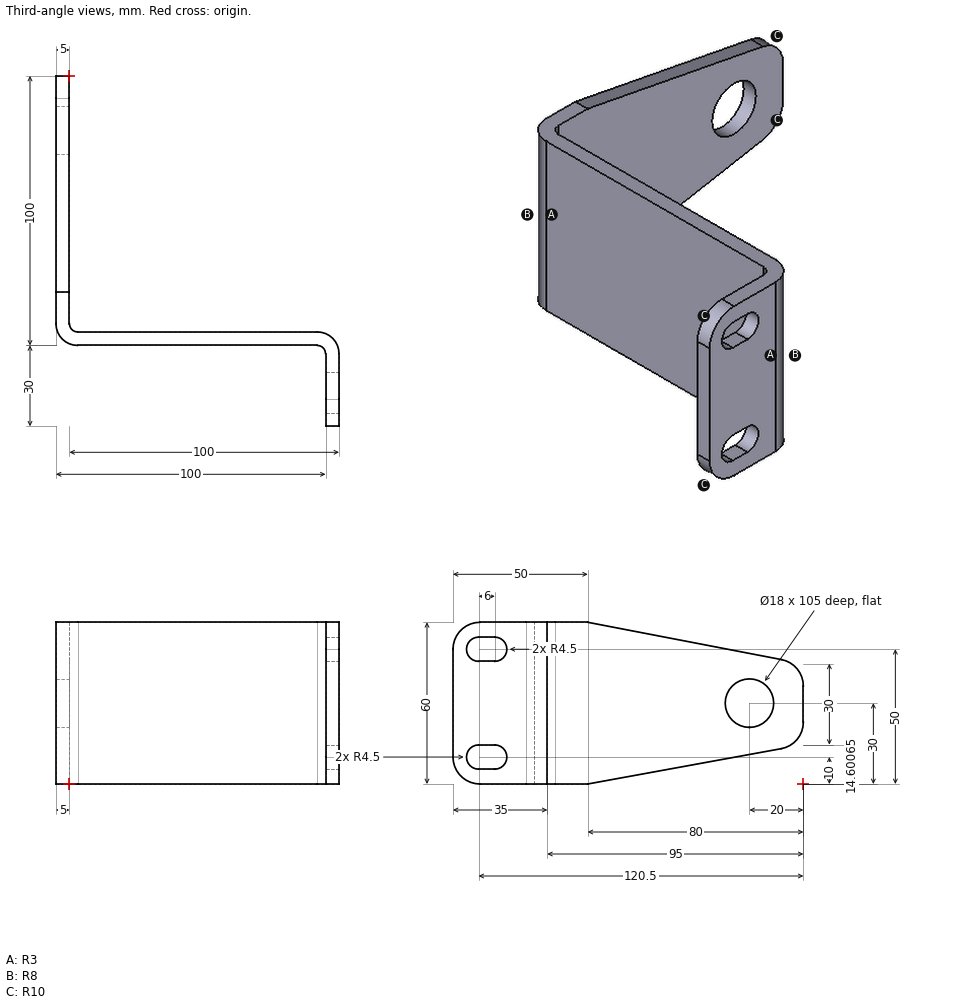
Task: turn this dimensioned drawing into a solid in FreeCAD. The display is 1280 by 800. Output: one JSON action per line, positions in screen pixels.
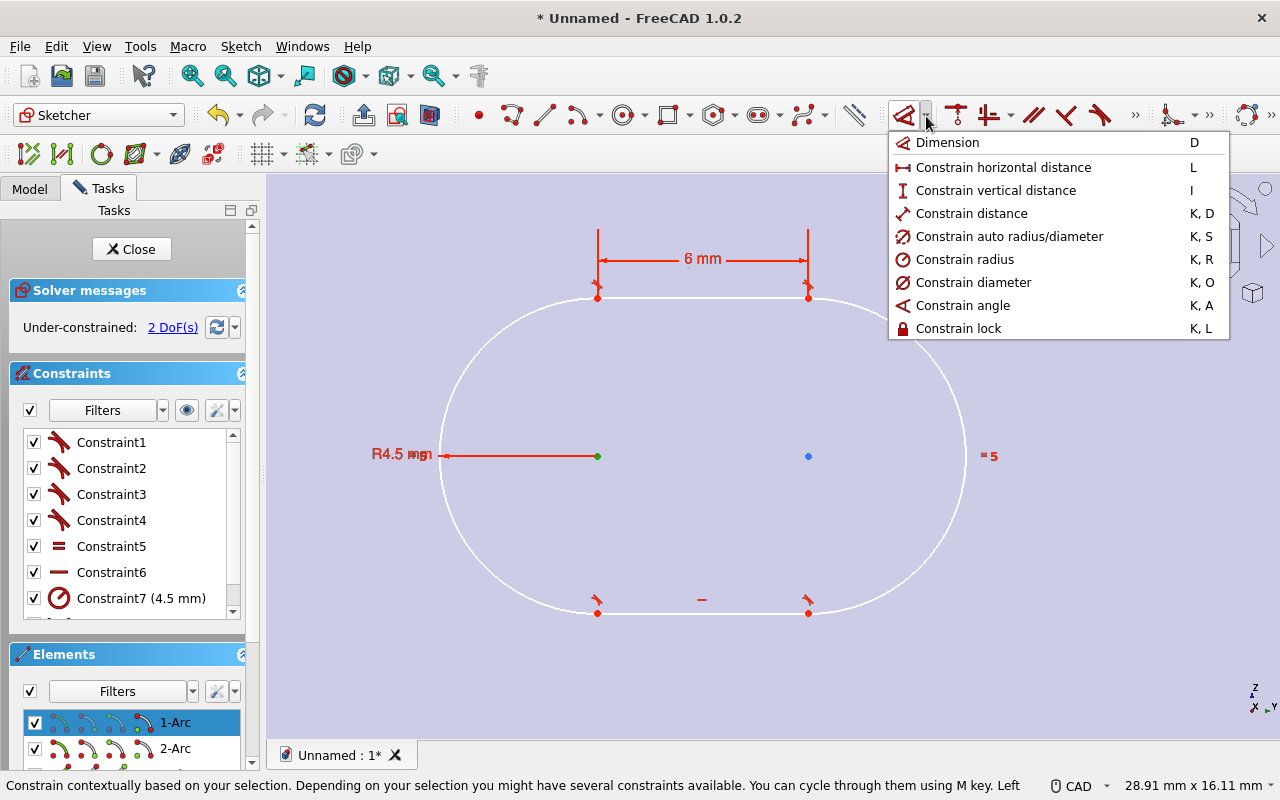
{"action": "left_click", "coordinate": [1059, 190]}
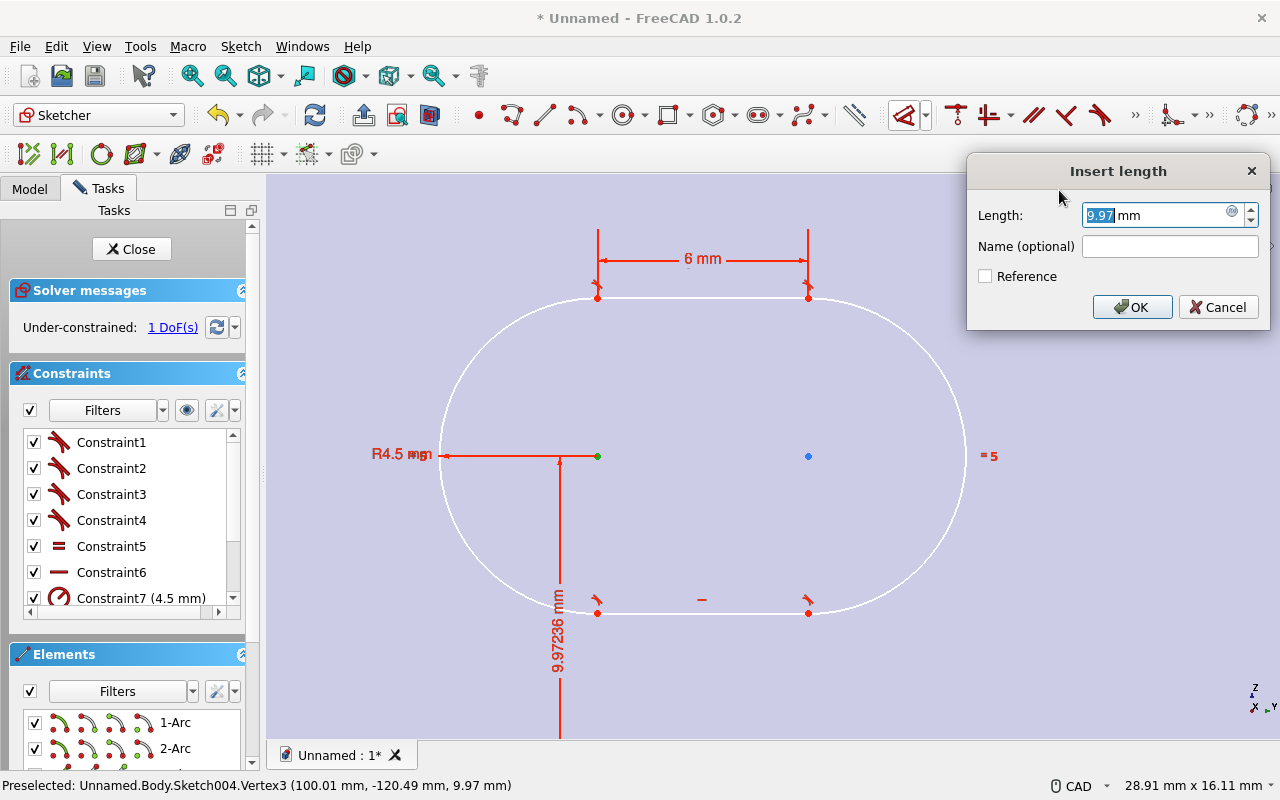
{"action": "type", "text": "10"}
{"action": "key", "text": "Return"}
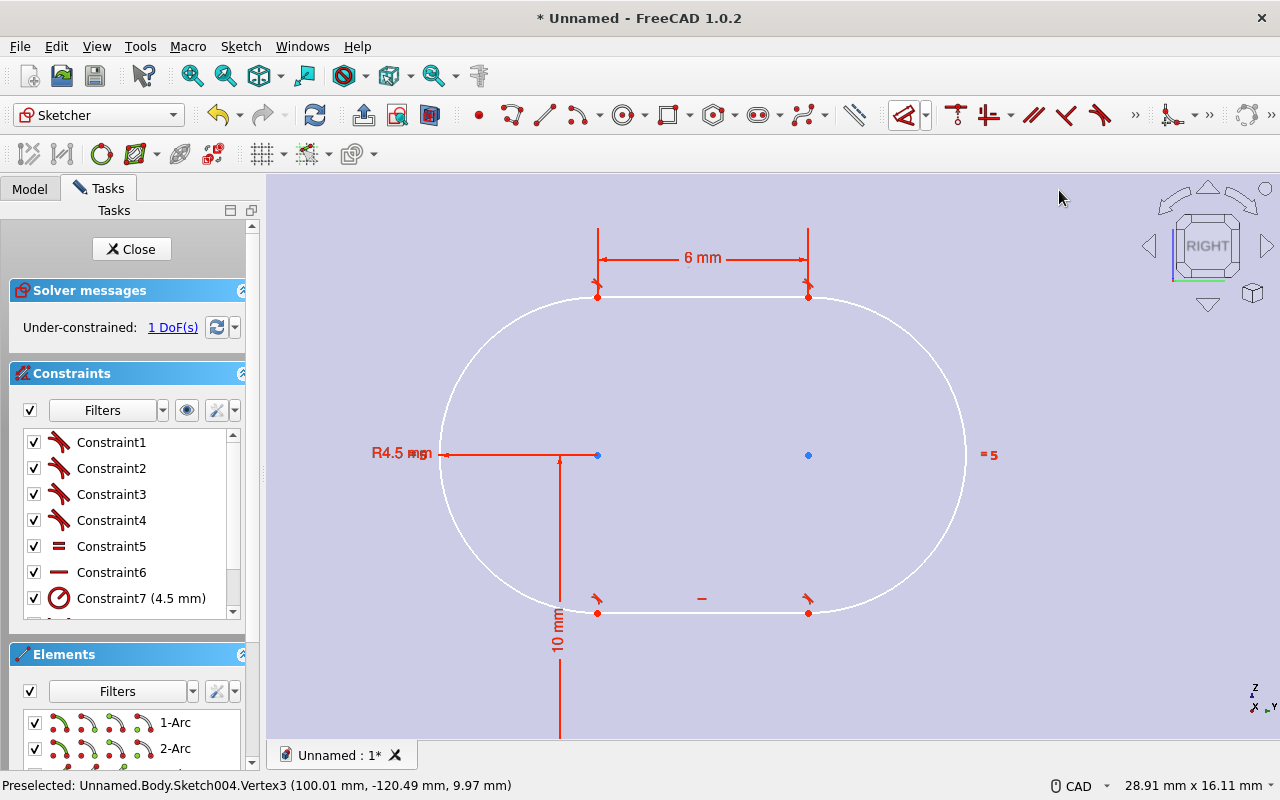
{"action": "left_click", "coordinate": [598, 297]}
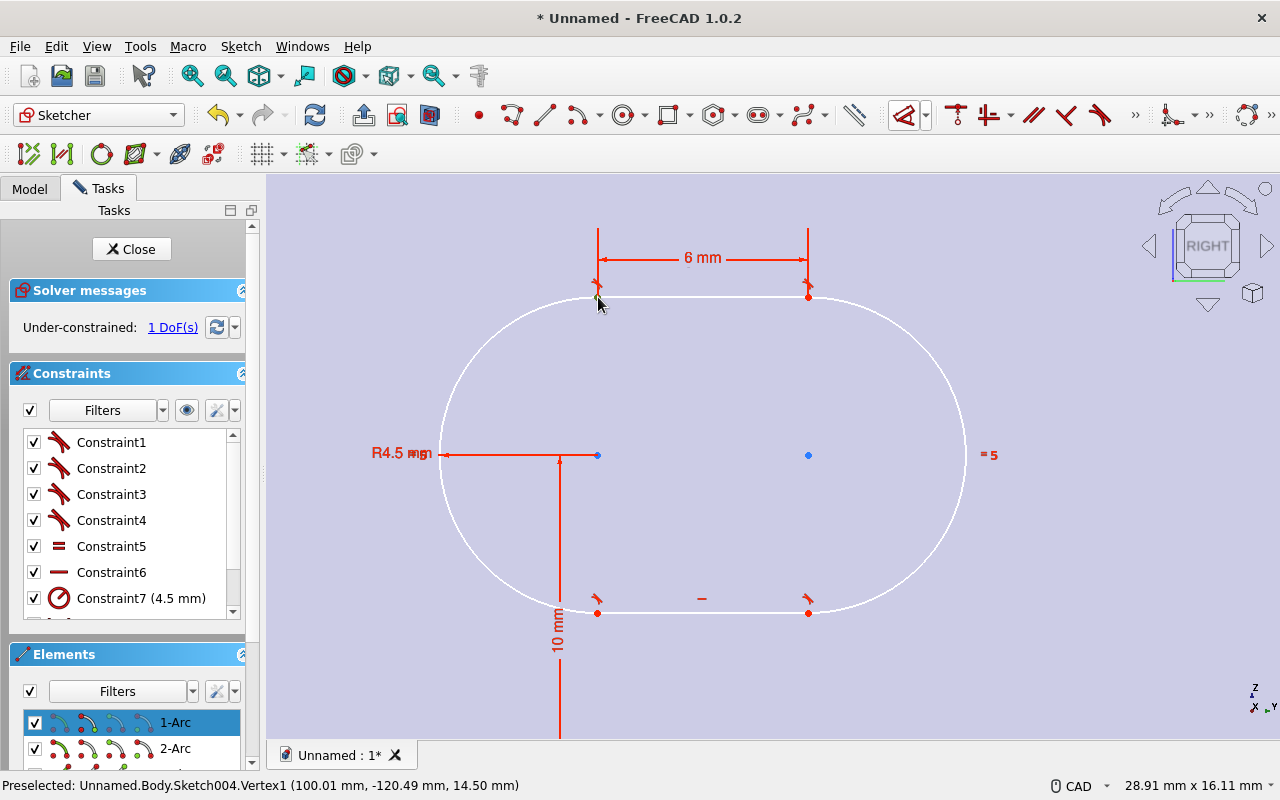
{"action": "left_click", "coordinate": [926, 116]}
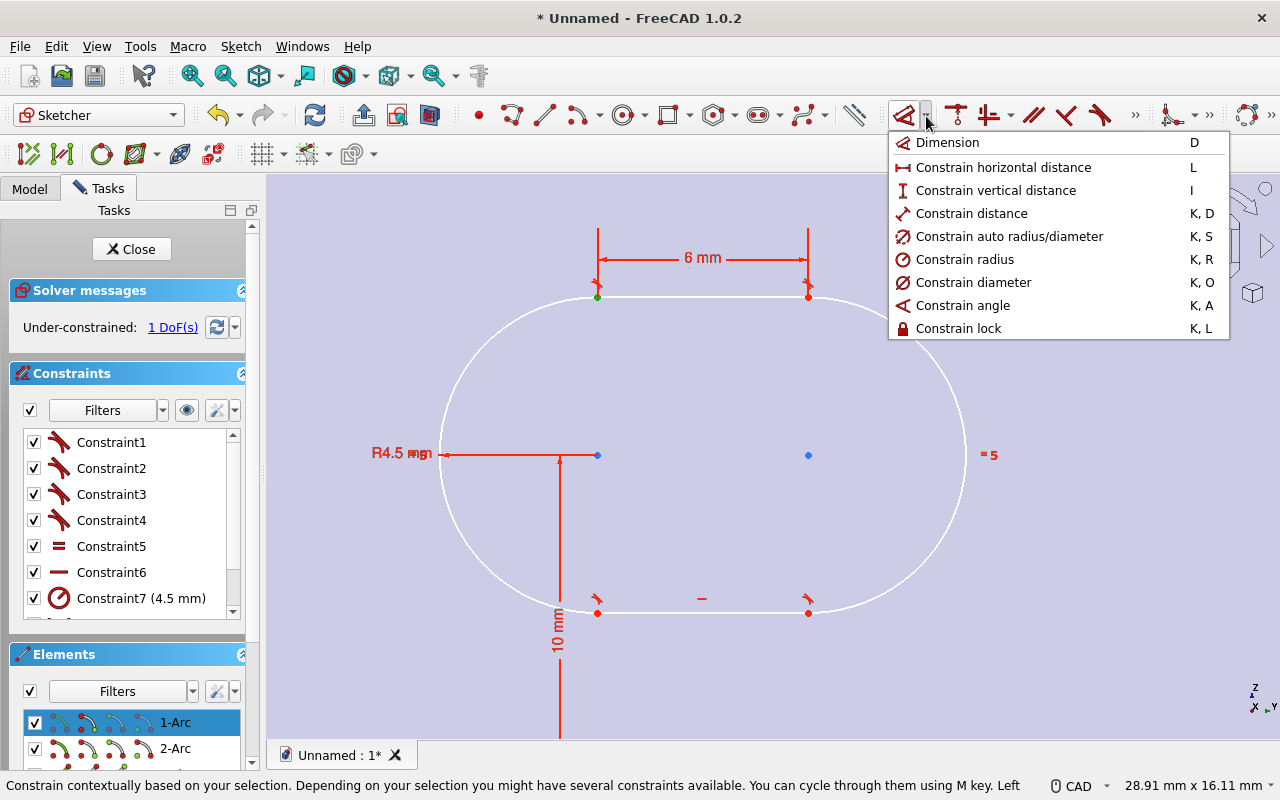
{"action": "left_click", "coordinate": [1059, 168]}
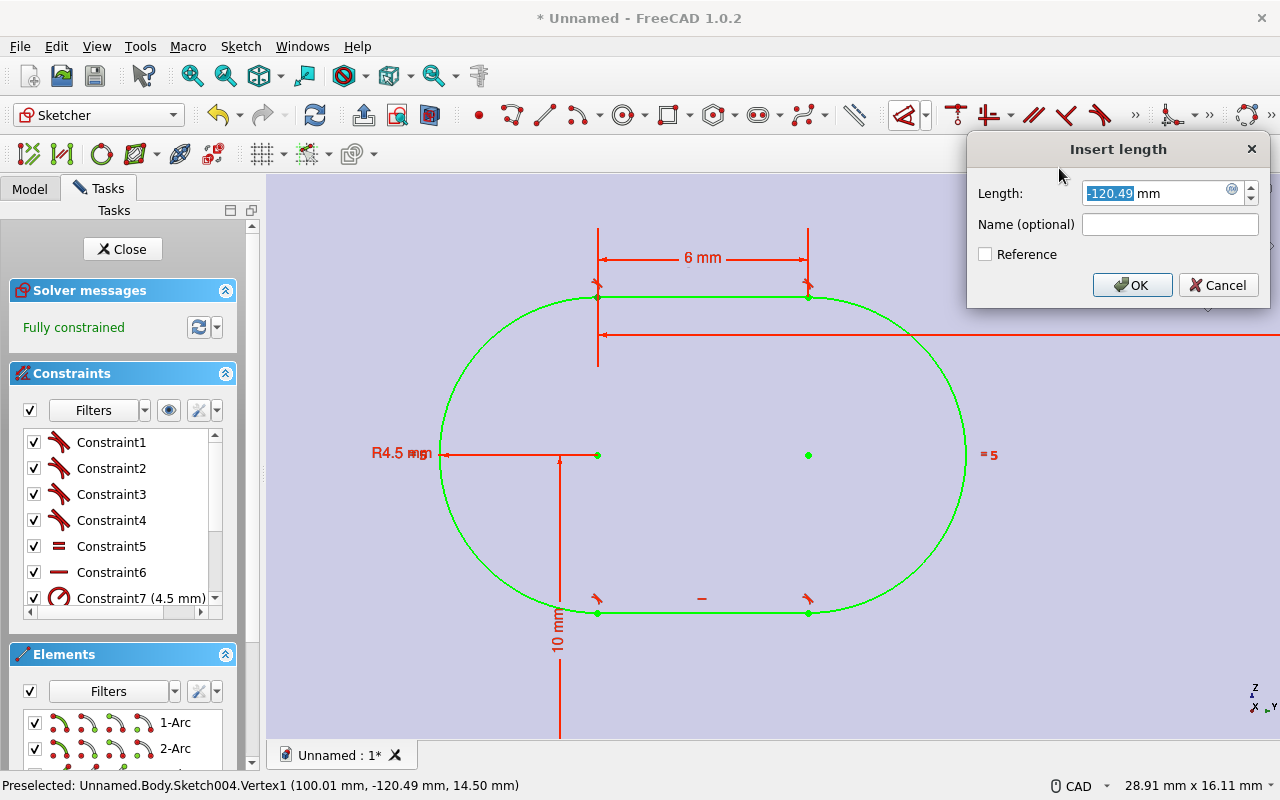
{"action": "type", "text": "-120.5"}
{"action": "key", "text": "Return"}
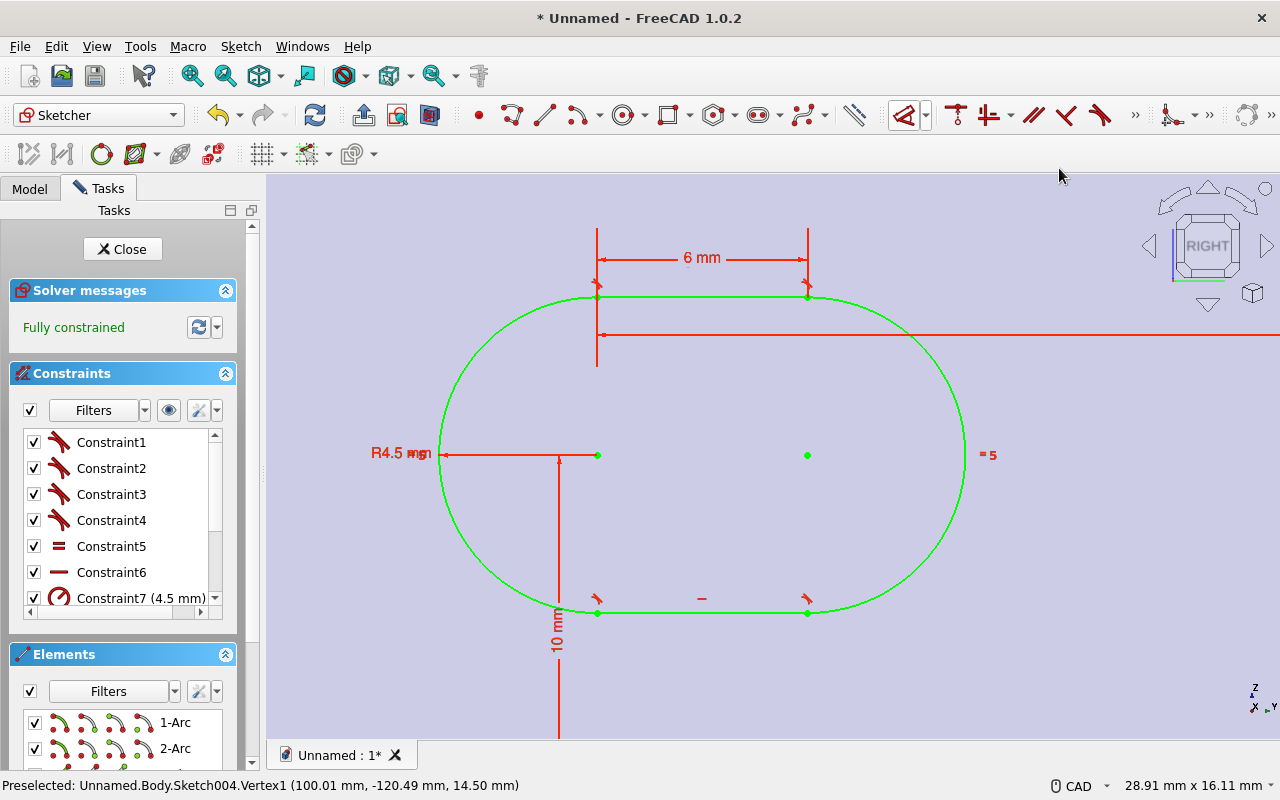
{"action": "left_click", "coordinate": [123, 249]}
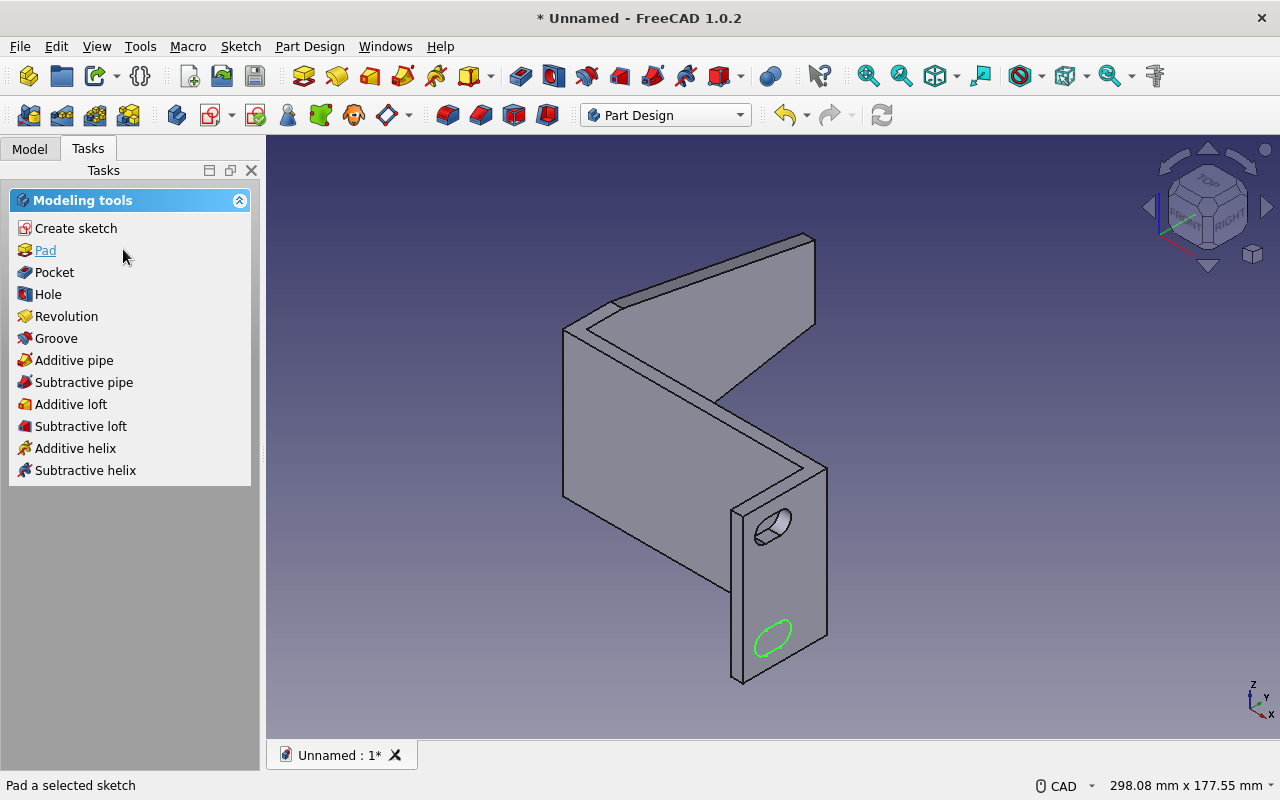
{"action": "left_click", "coordinate": [521, 76]}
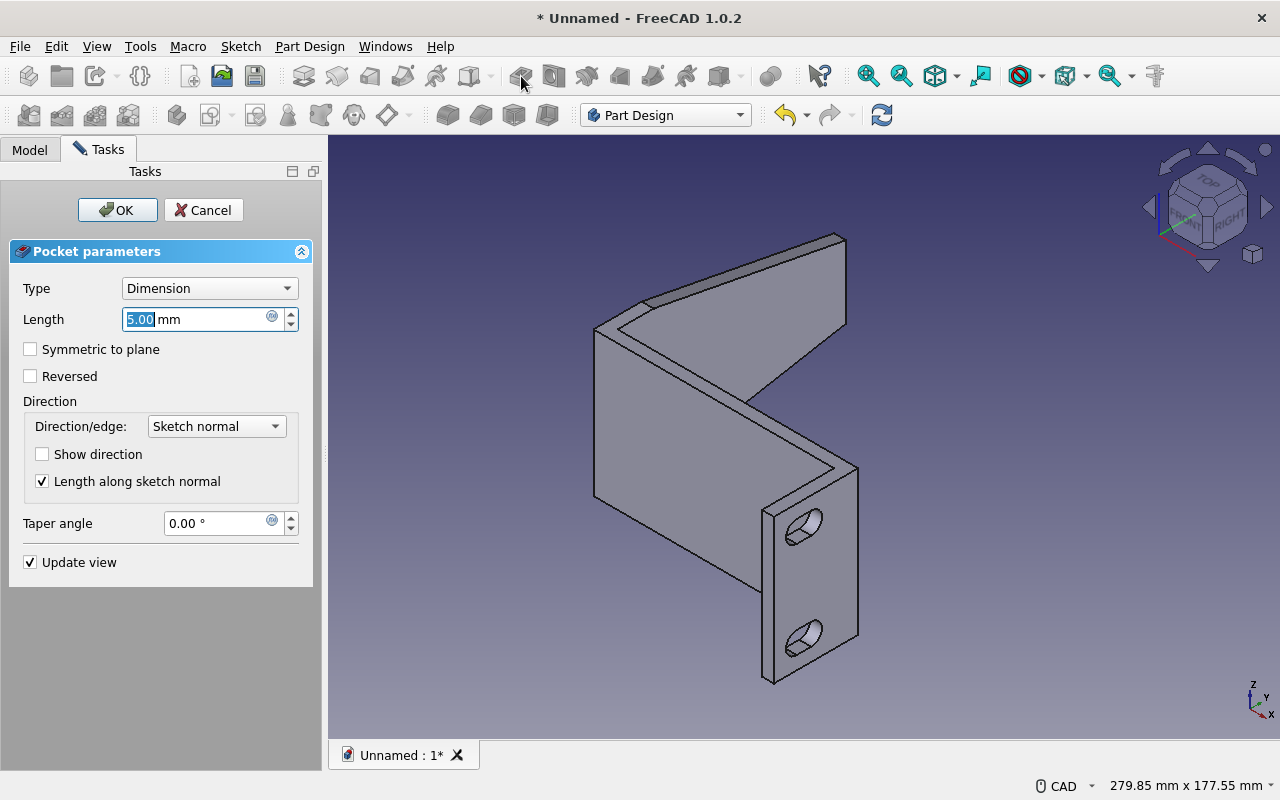
{"action": "left_click", "coordinate": [210, 288]}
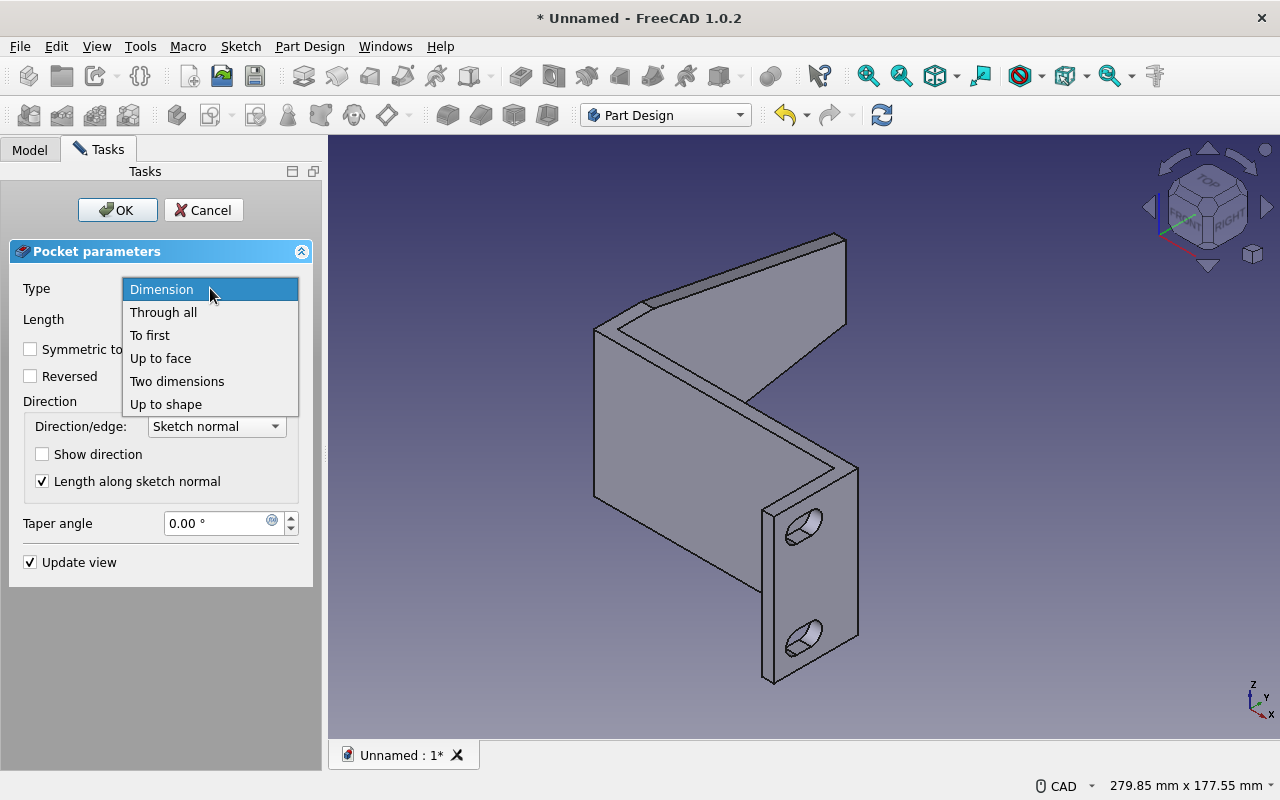
{"action": "left_click", "coordinate": [208, 312]}